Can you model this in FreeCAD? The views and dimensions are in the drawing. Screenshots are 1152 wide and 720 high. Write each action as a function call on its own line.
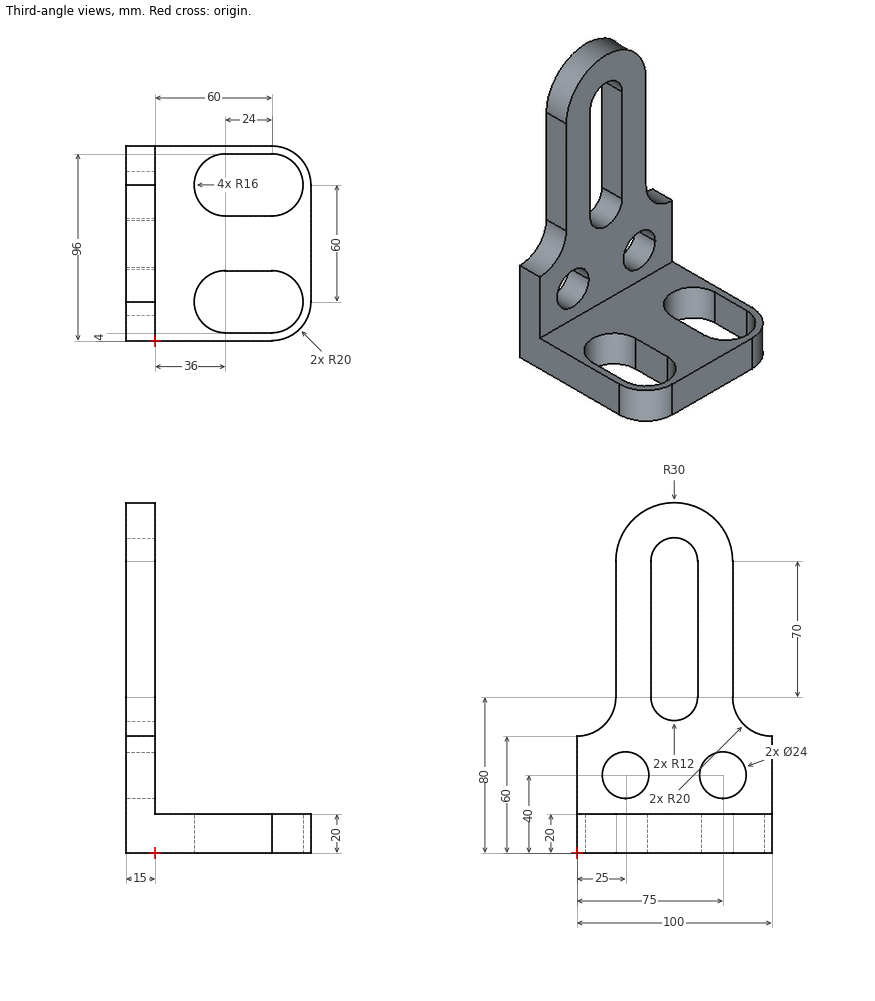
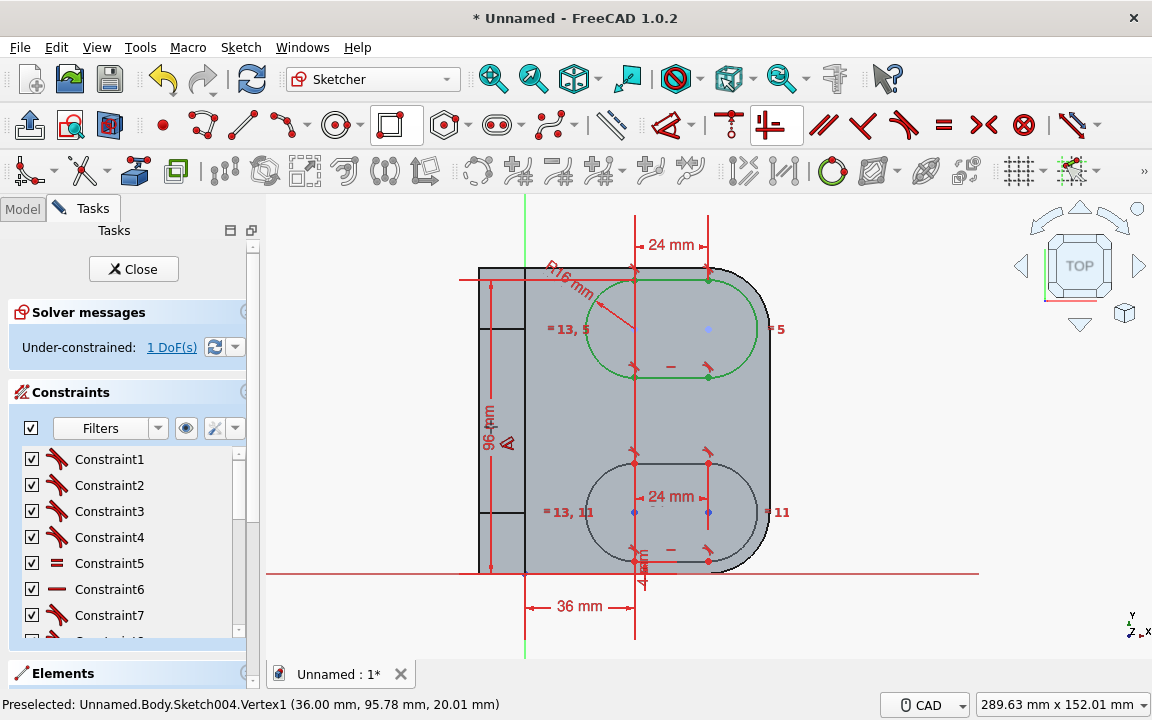
click(635, 464)
click(580, 430)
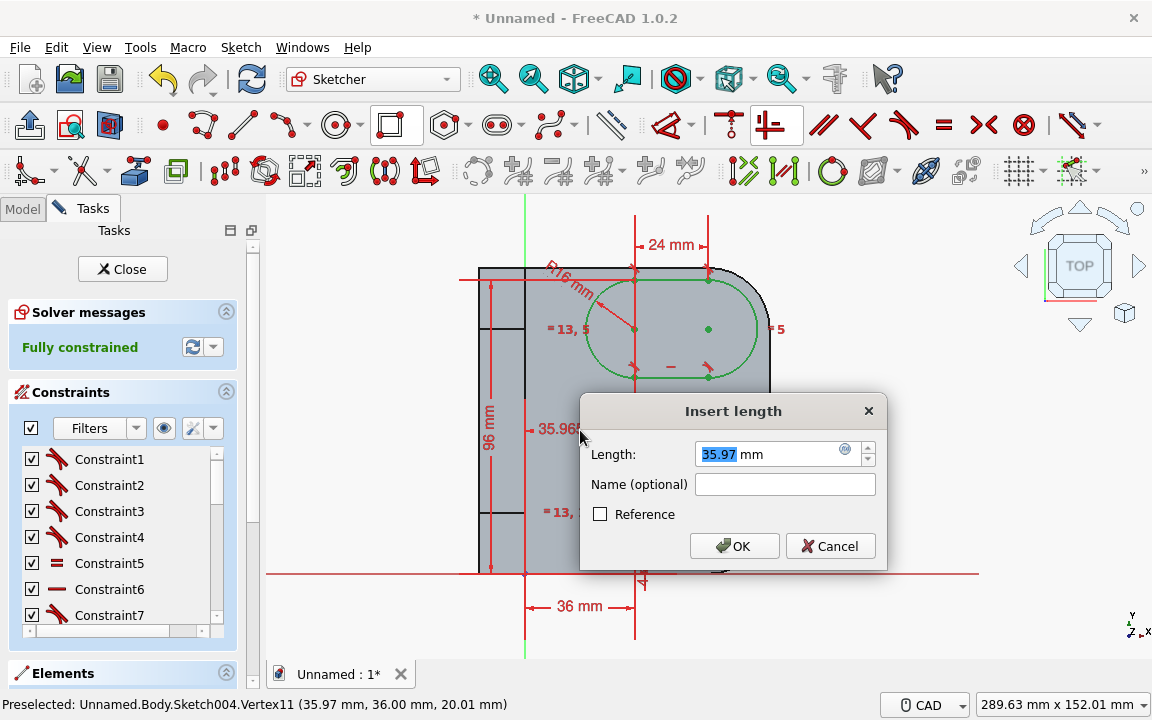
text(36)
key(Return)
key(Escape)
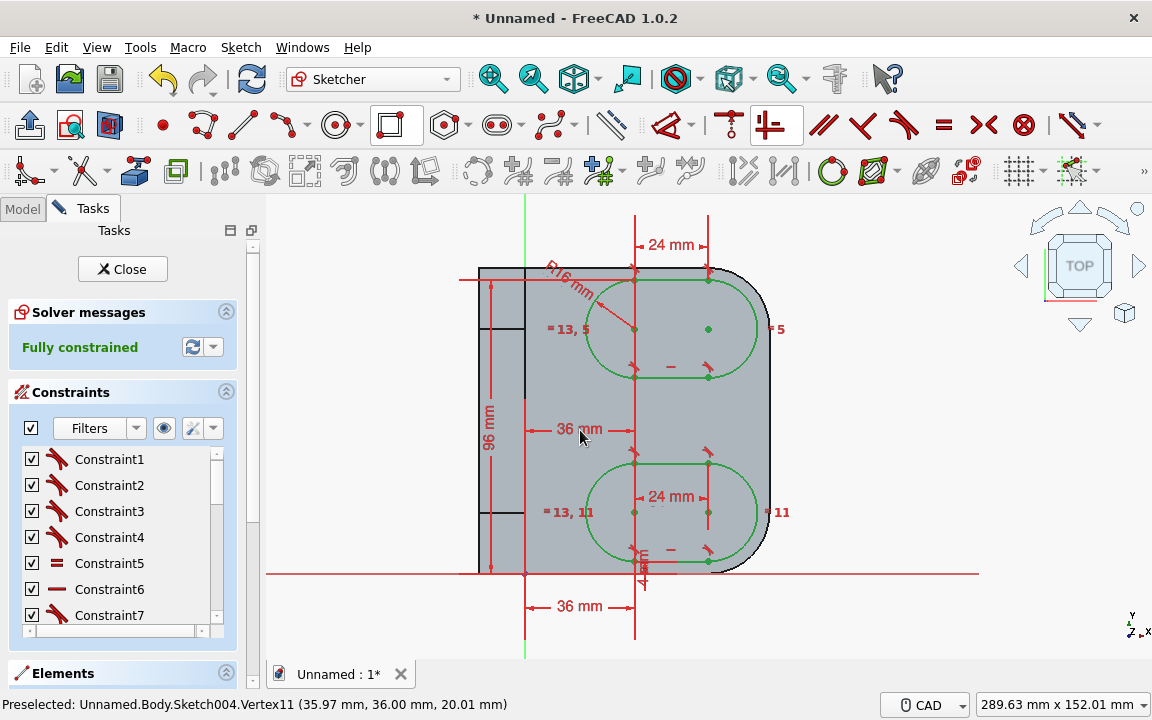
click(123, 269)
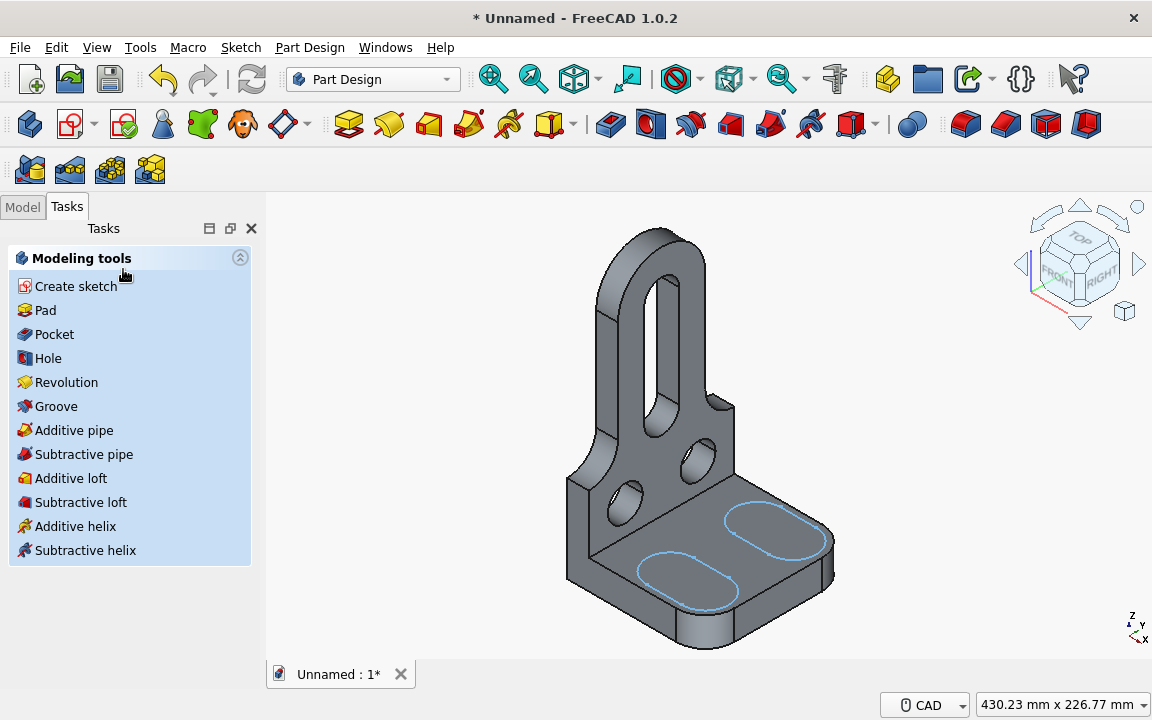
click(612, 124)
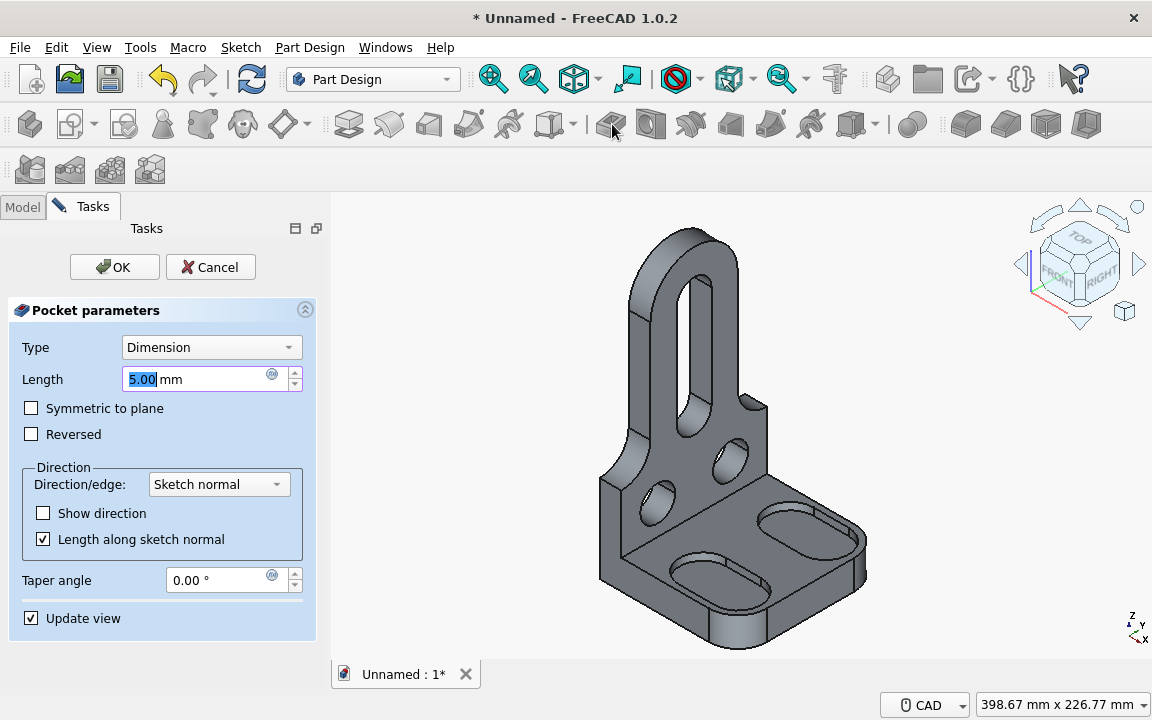
text(20)
key(Tab)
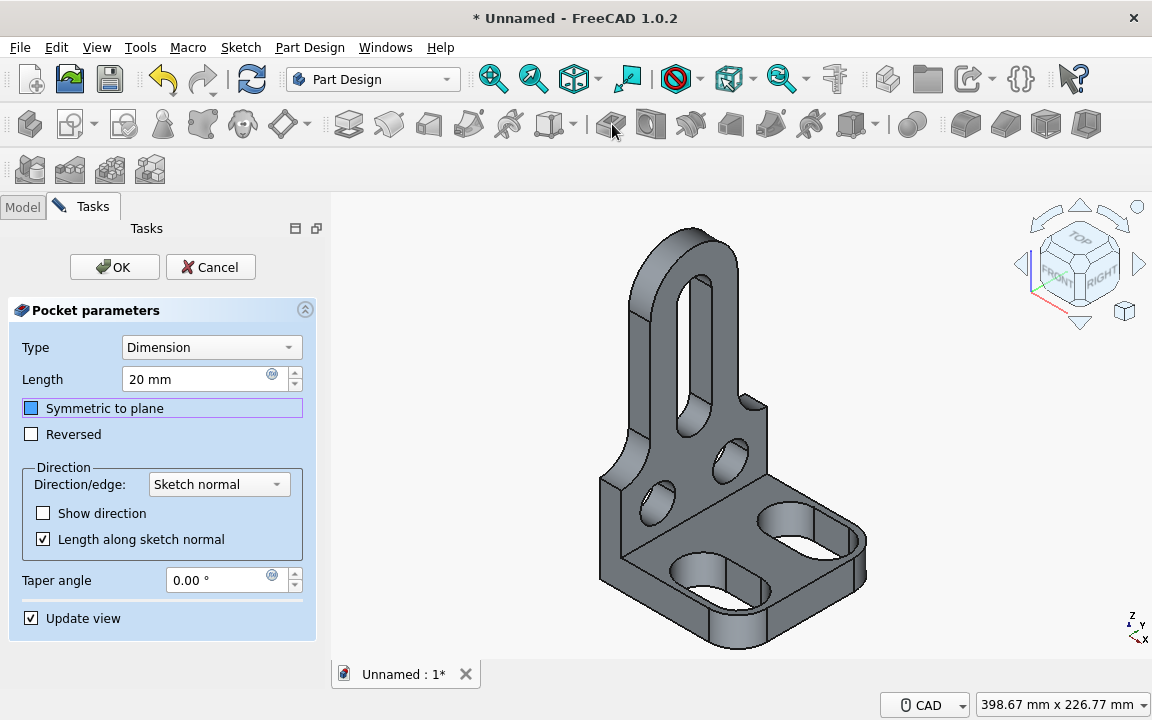
click(115, 267)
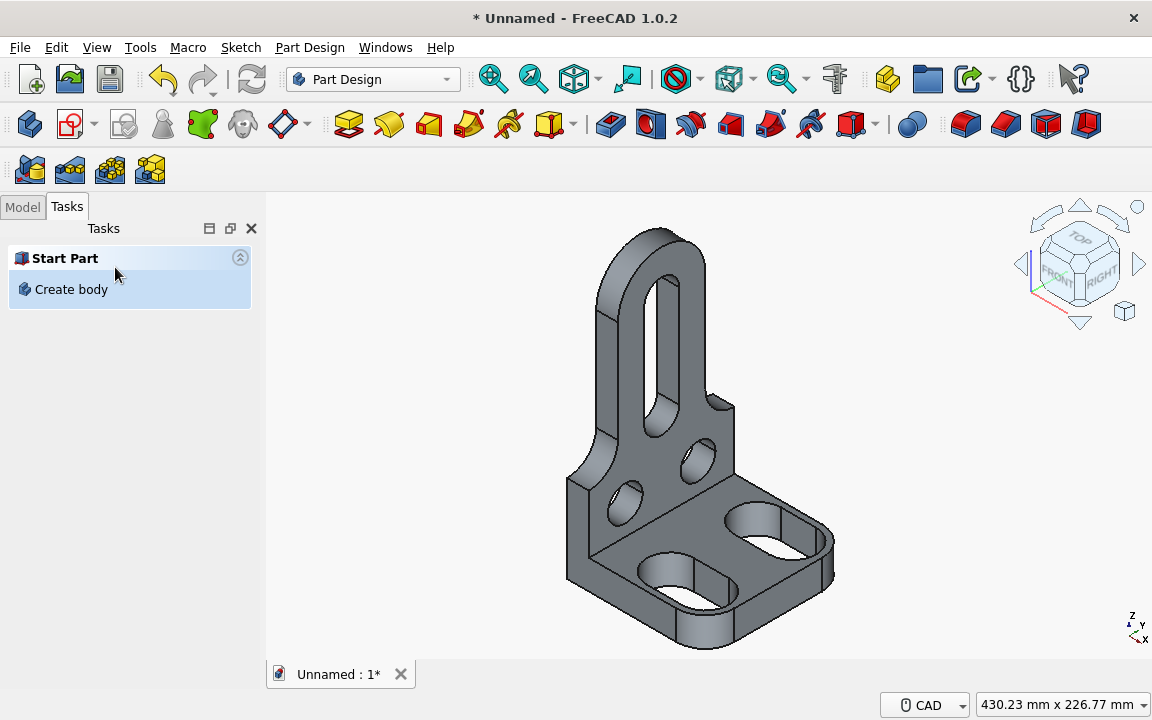
click(494, 80)